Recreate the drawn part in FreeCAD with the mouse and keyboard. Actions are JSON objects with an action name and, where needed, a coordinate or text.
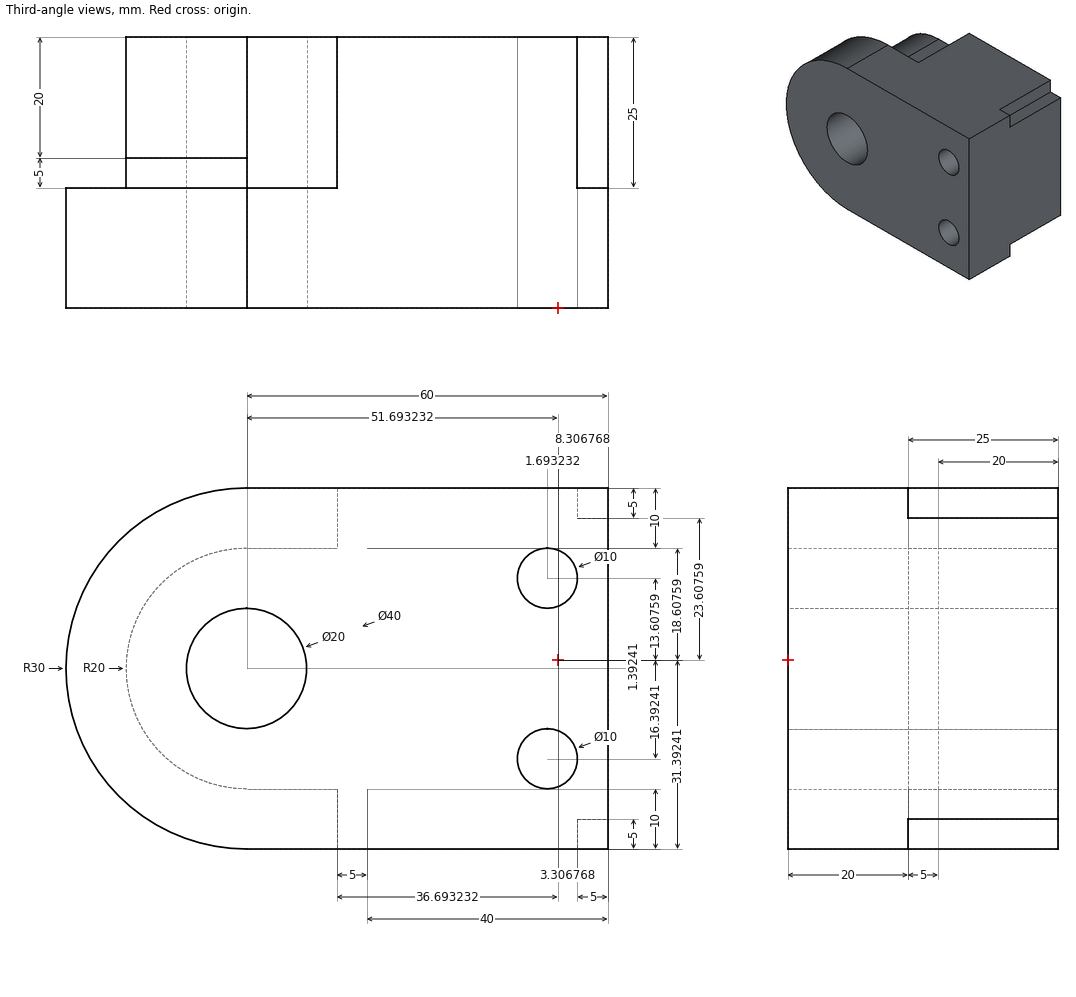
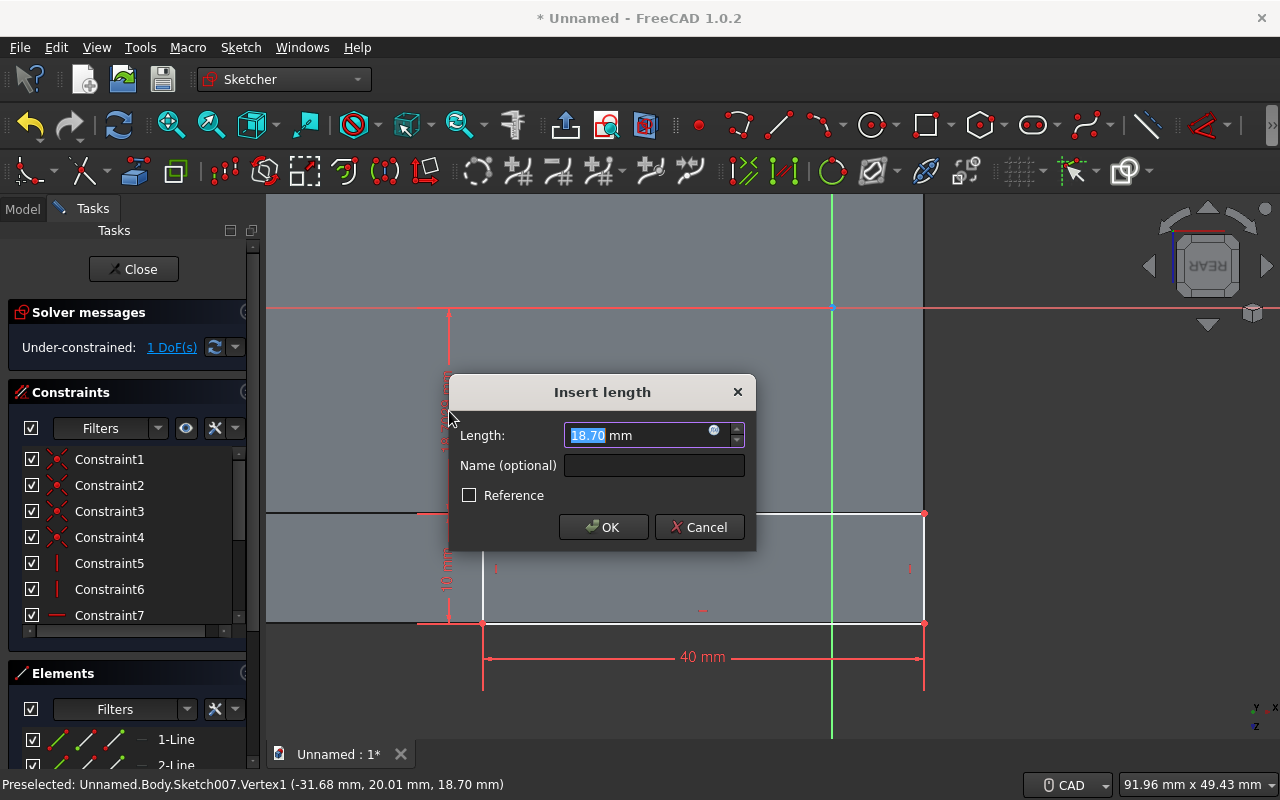
{"action": "type", "text": "18.60759"}
{"action": "key", "text": "Return"}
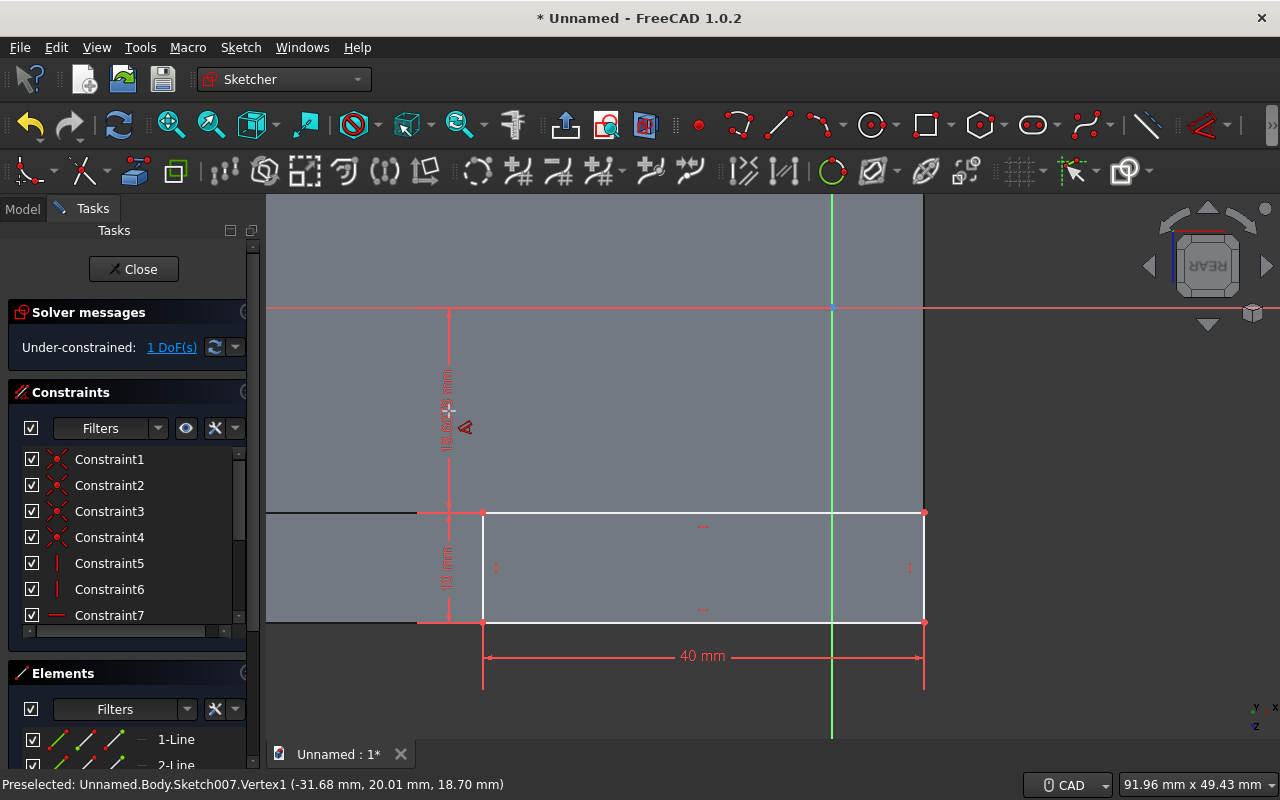
{"action": "left_click", "coordinate": [924, 623]}
{"action": "left_click", "coordinate": [878, 657]}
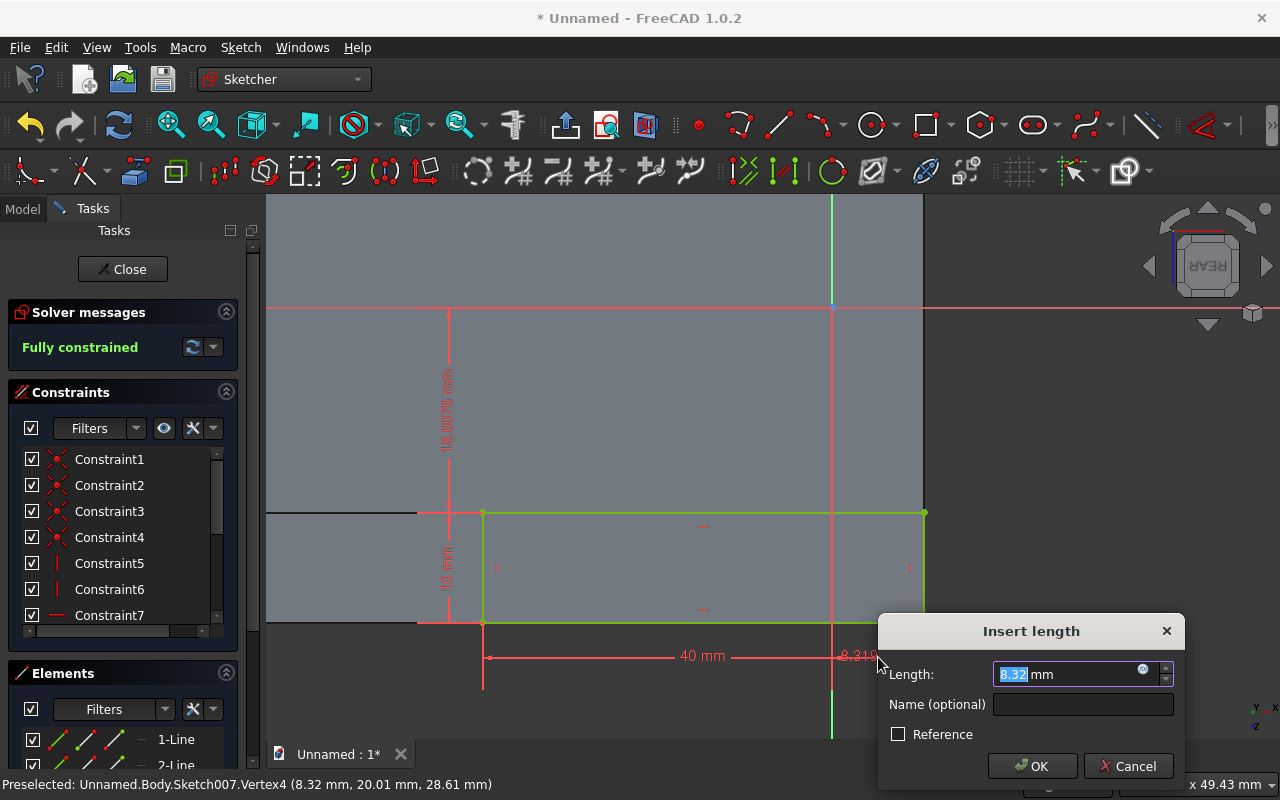
{"action": "type", "text": "8.306768"}
{"action": "key", "text": "Return"}
{"action": "key", "text": "Escape"}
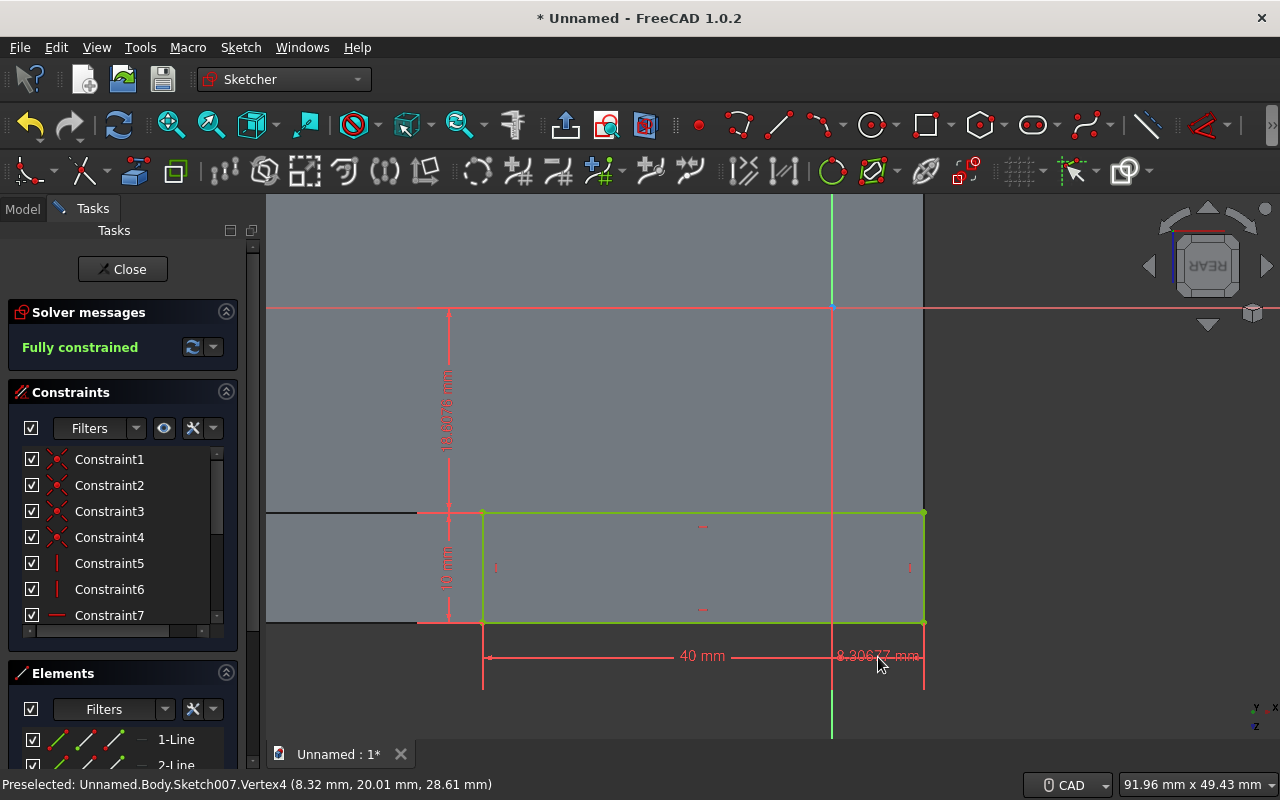
{"action": "left_click", "coordinate": [123, 269]}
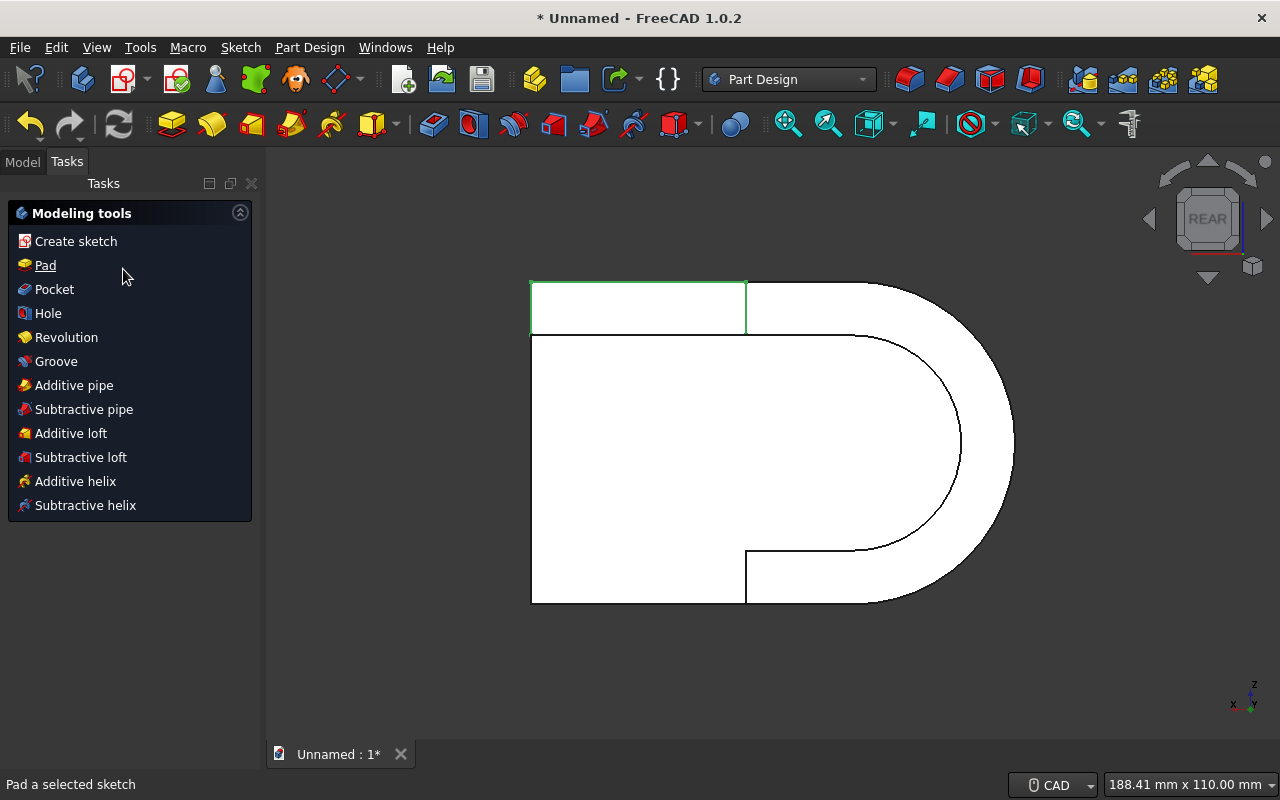
{"action": "left_click", "coordinate": [172, 124]}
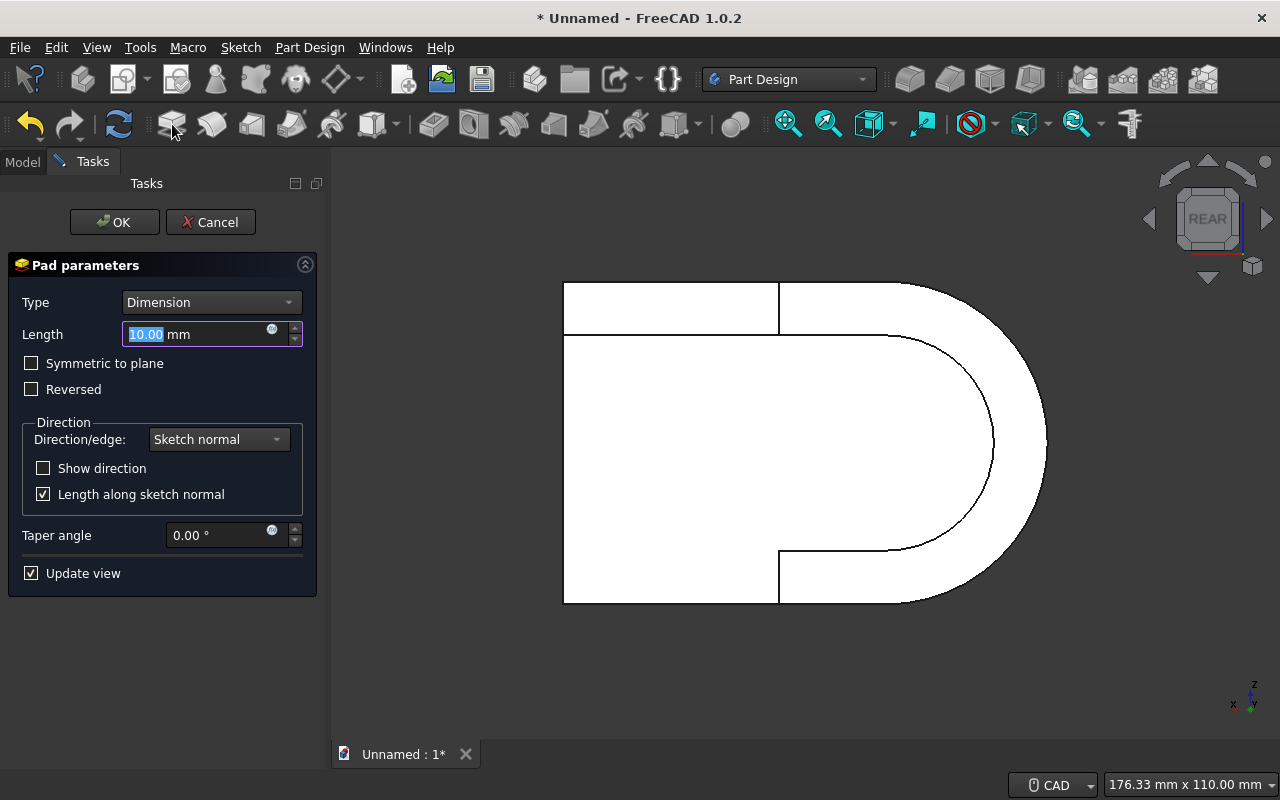
{"action": "type", "text": "5"}
{"action": "key", "text": "Tab"}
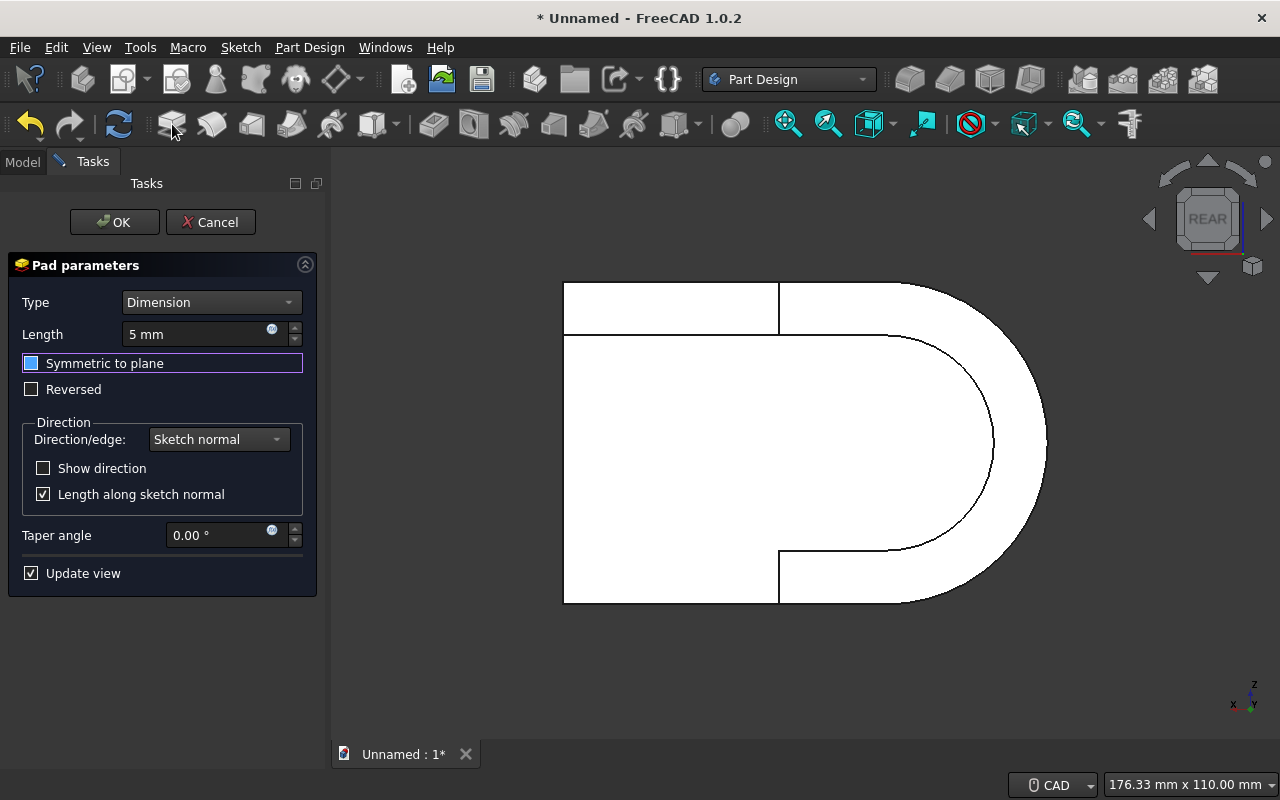
{"action": "left_click", "coordinate": [115, 222]}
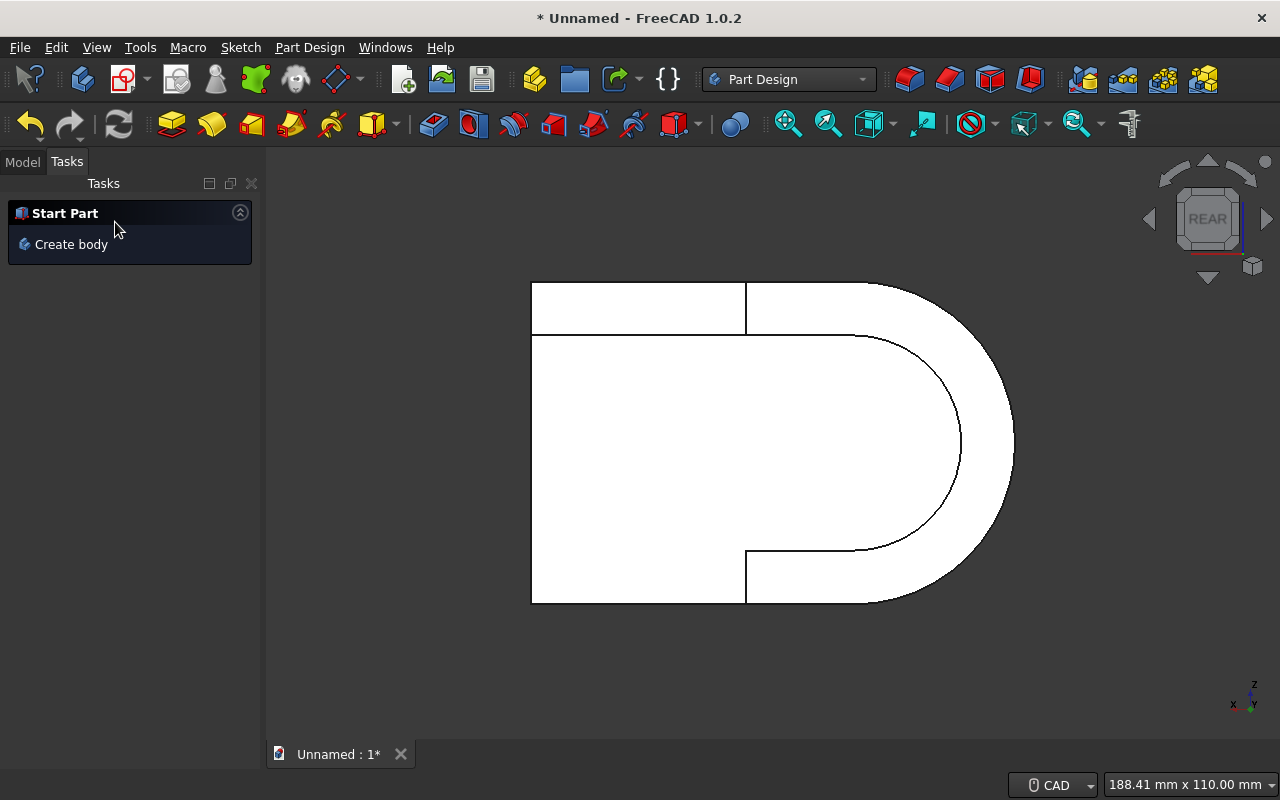
{"action": "left_click", "coordinate": [577, 307]}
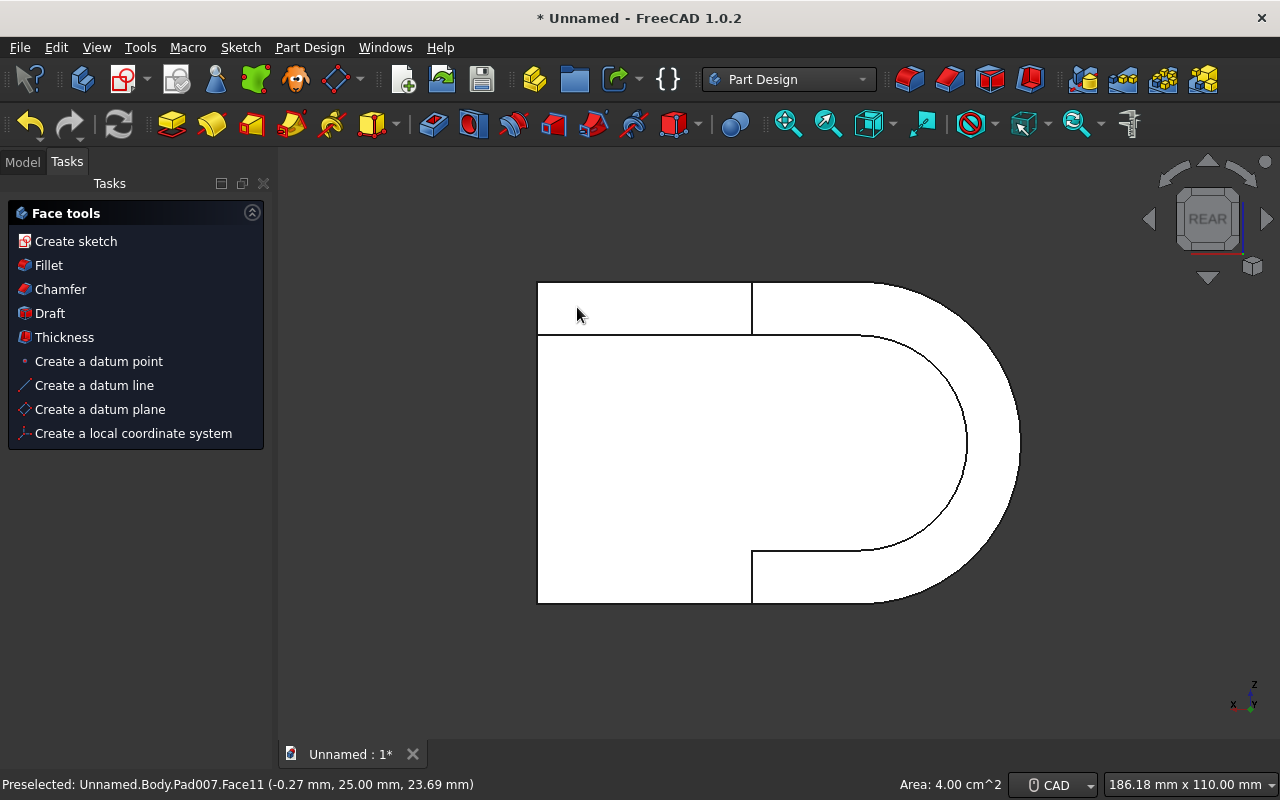
{"action": "left_click", "coordinate": [124, 80]}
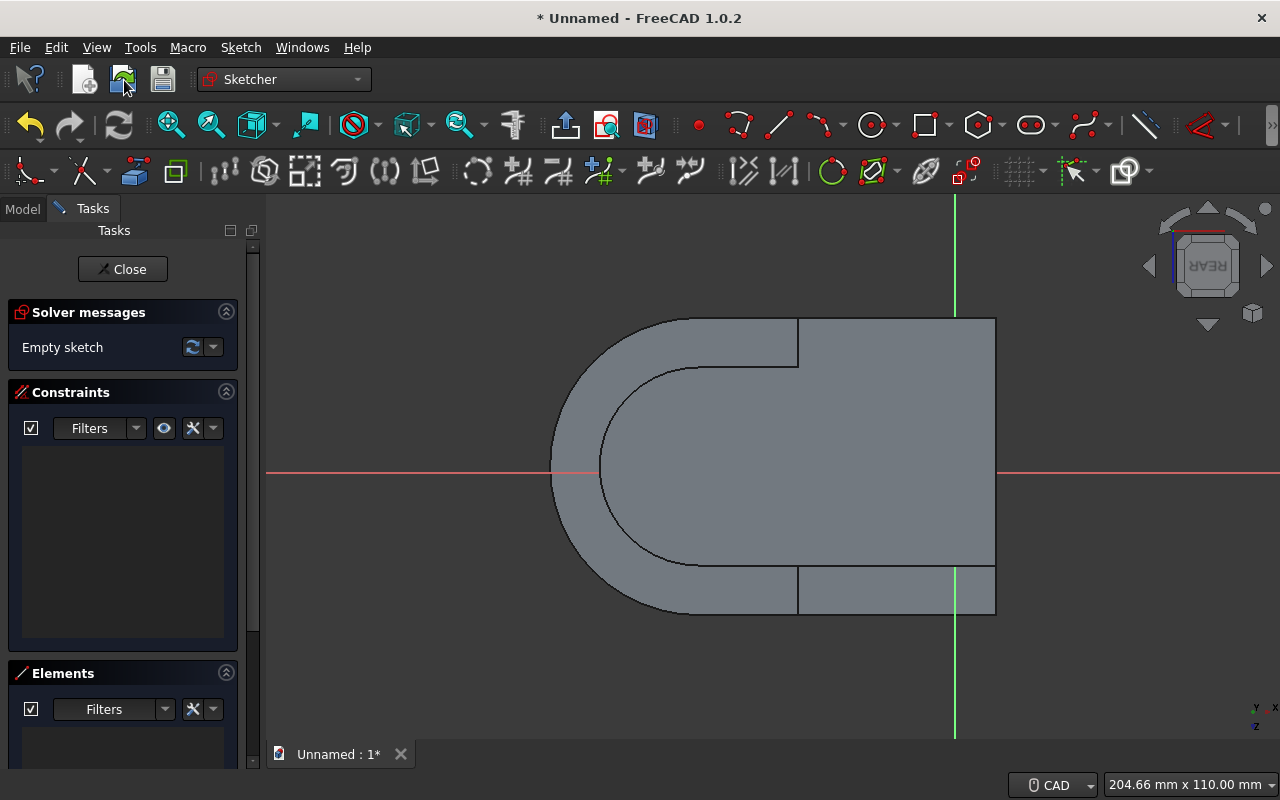
{"action": "key", "text": "q s"}